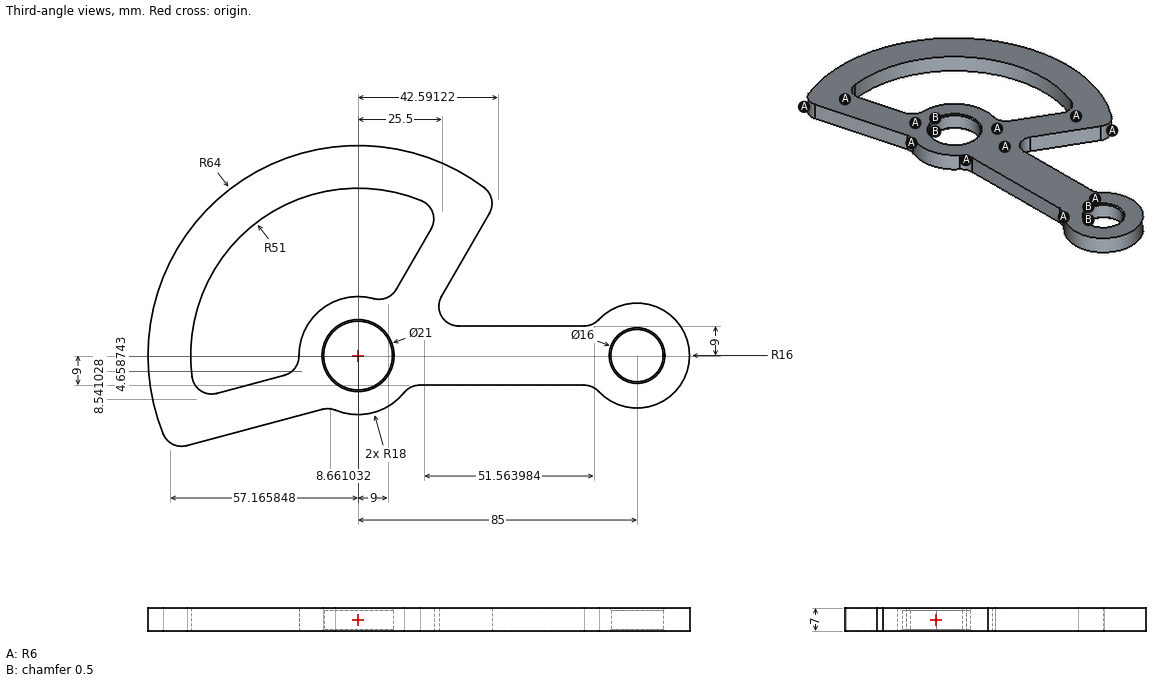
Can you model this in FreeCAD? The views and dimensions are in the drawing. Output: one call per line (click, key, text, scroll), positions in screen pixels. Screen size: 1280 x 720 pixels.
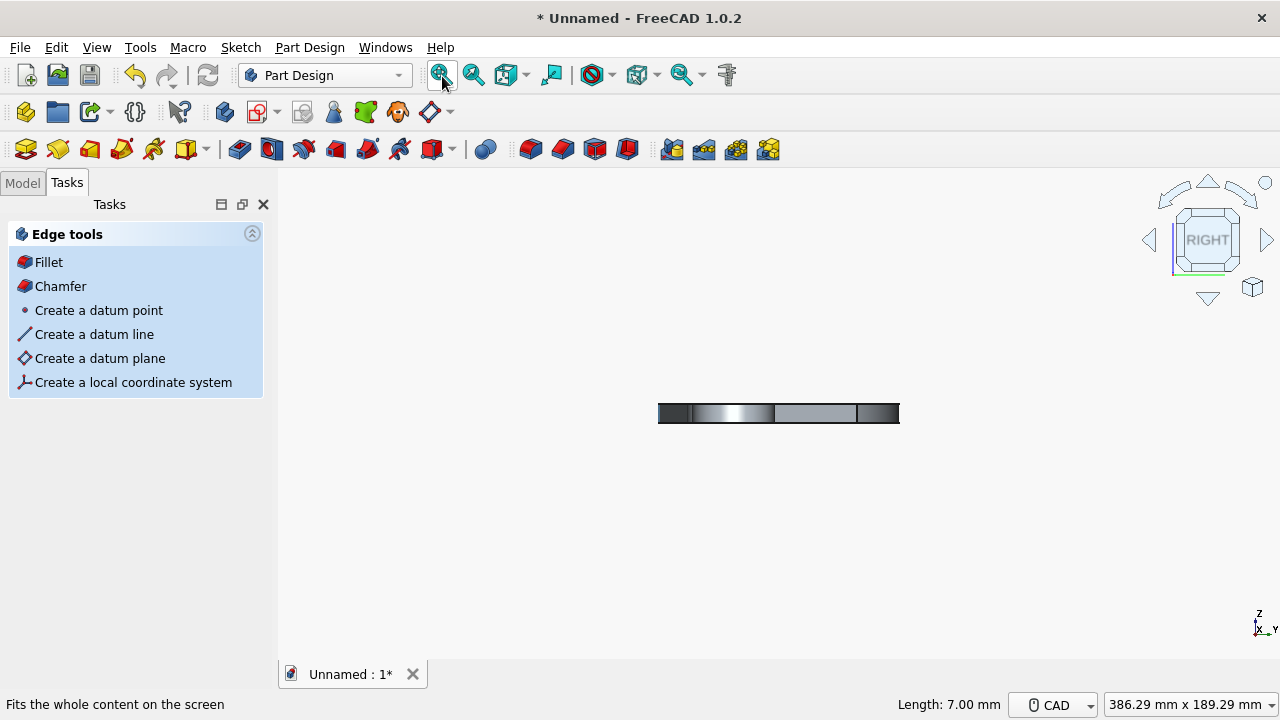
click(857, 412, ctrl)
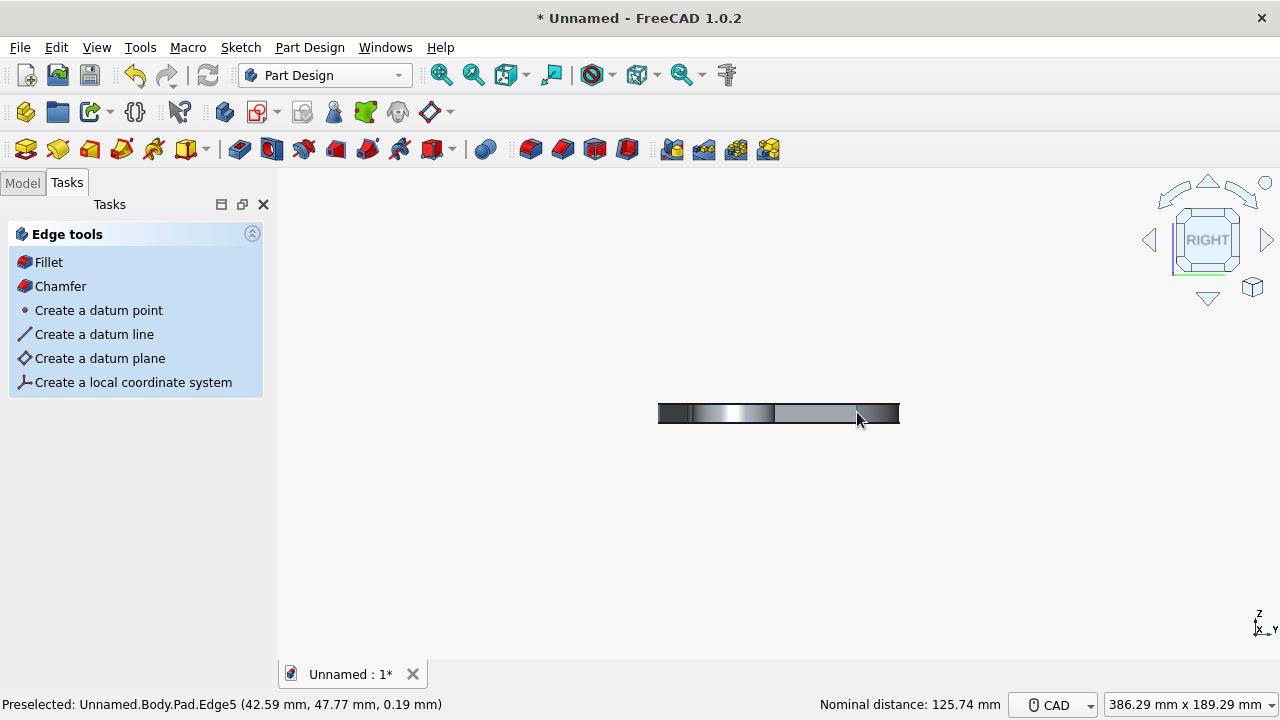
scroll(710, 412, up, 4)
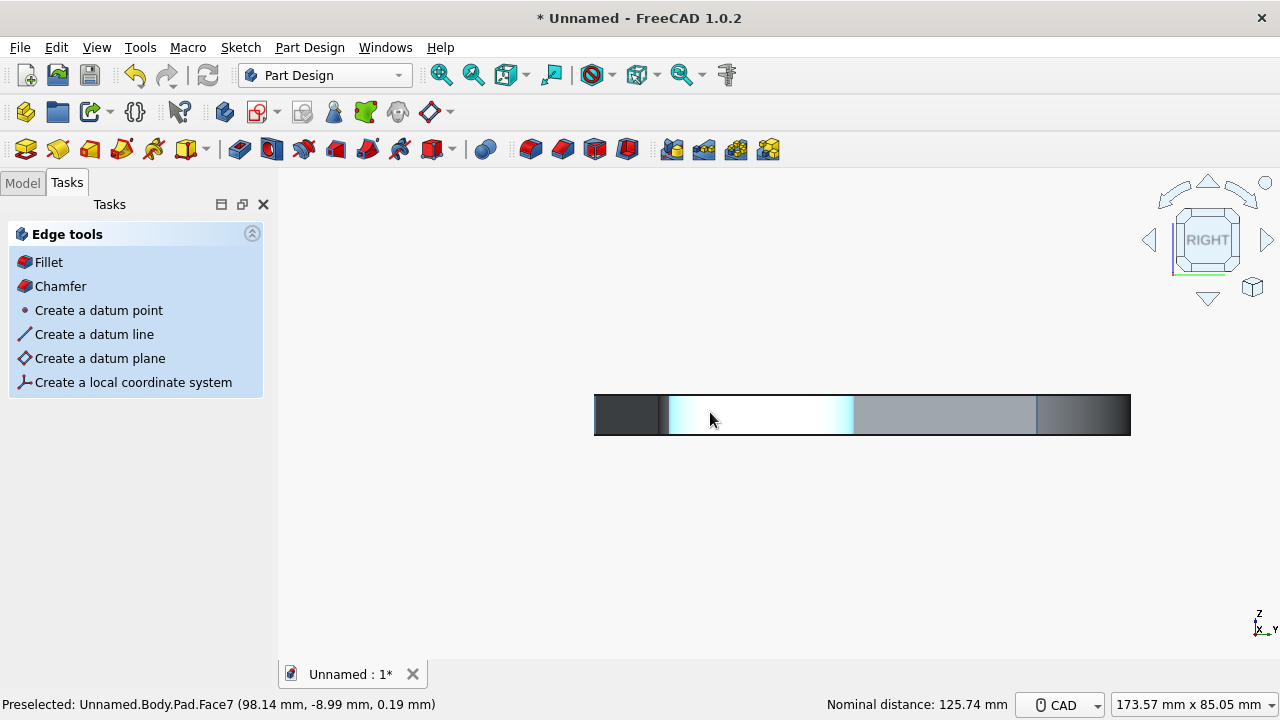
click(442, 76)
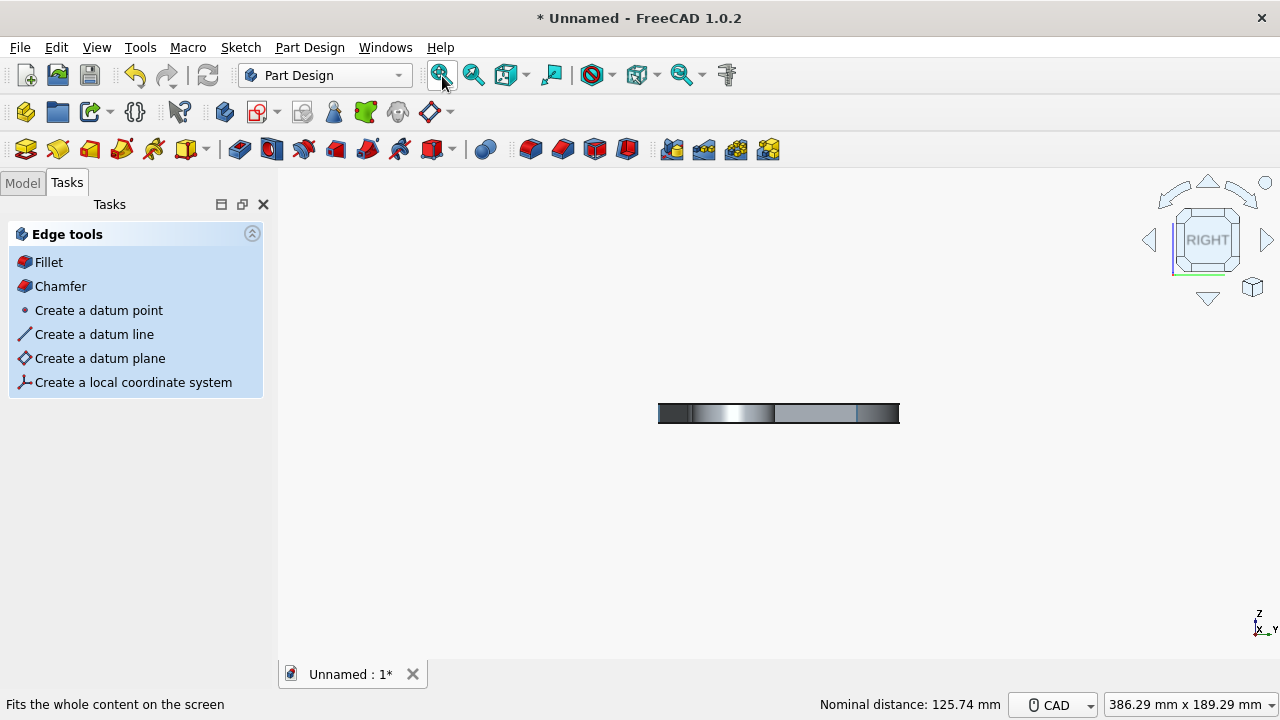
key(5)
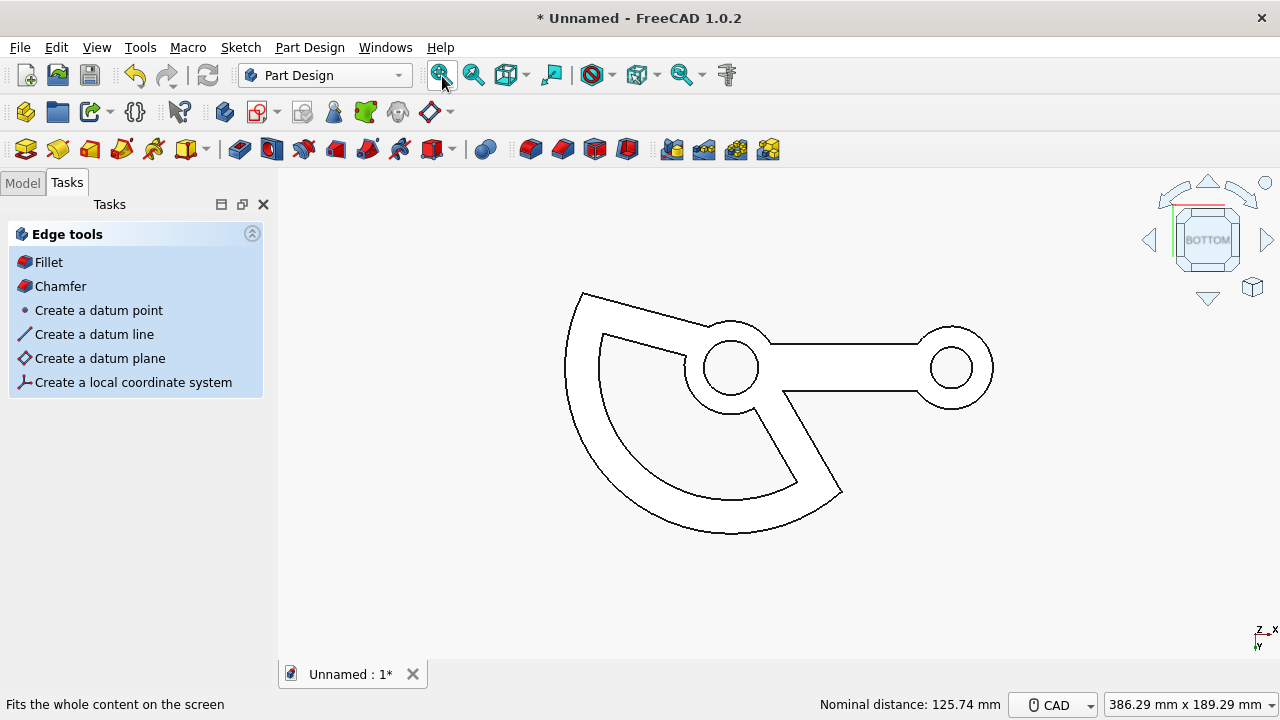
scroll(917, 343, up, 4)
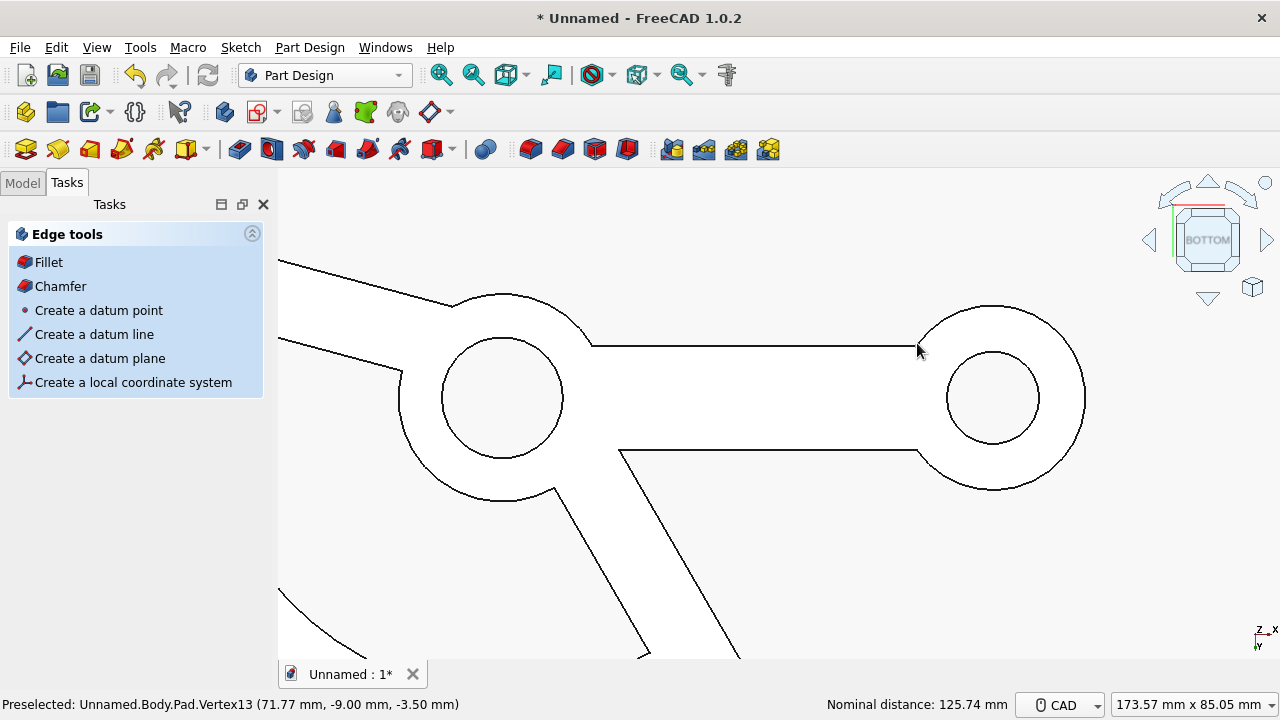
click(442, 76)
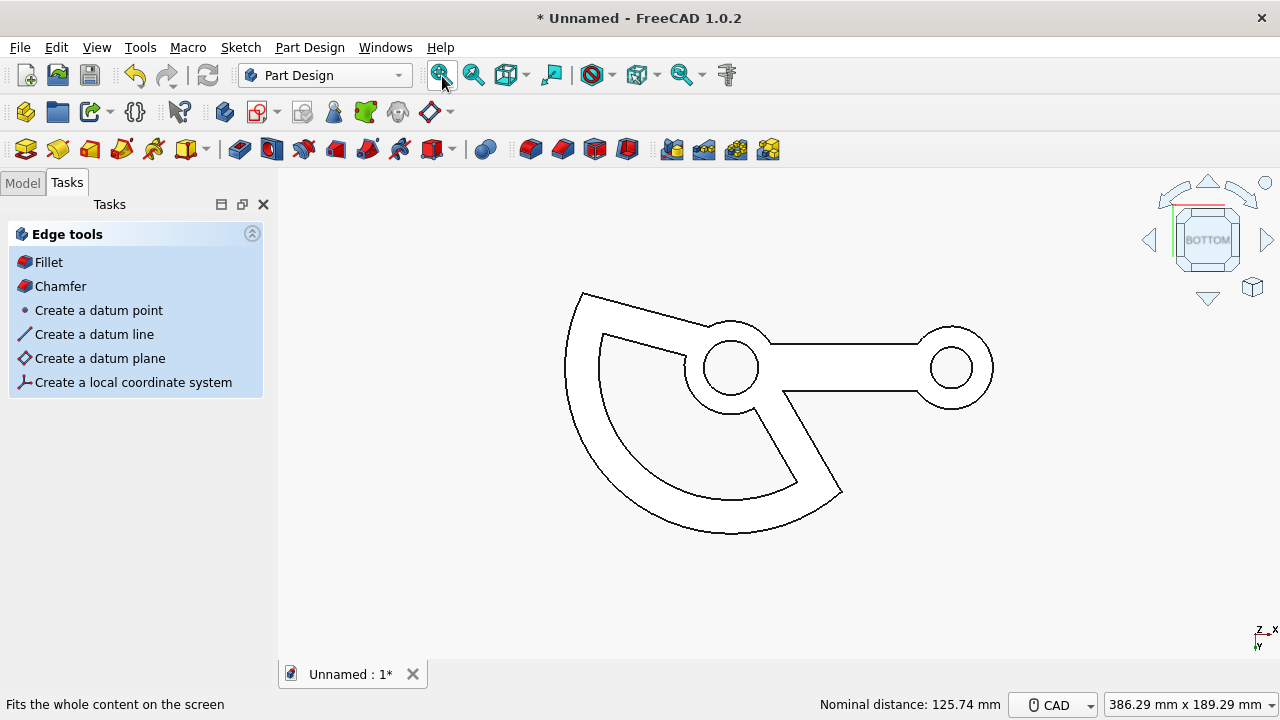
key(4)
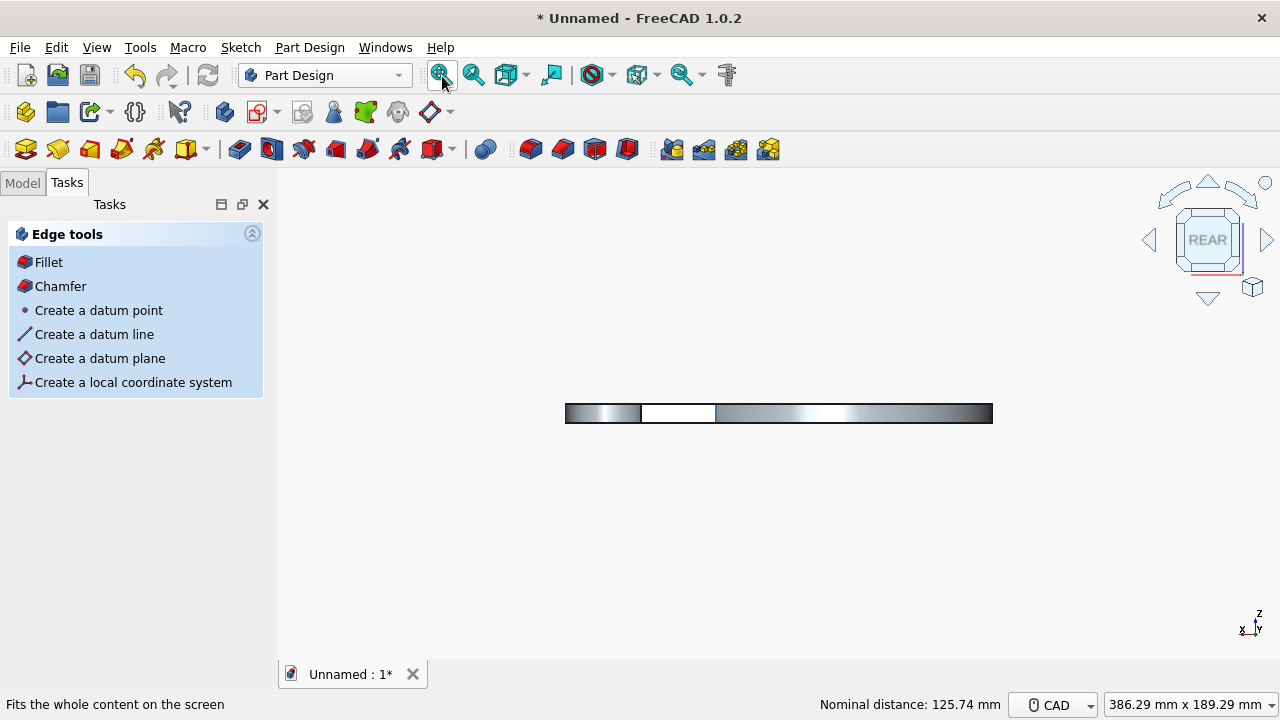
key(v)
key(f)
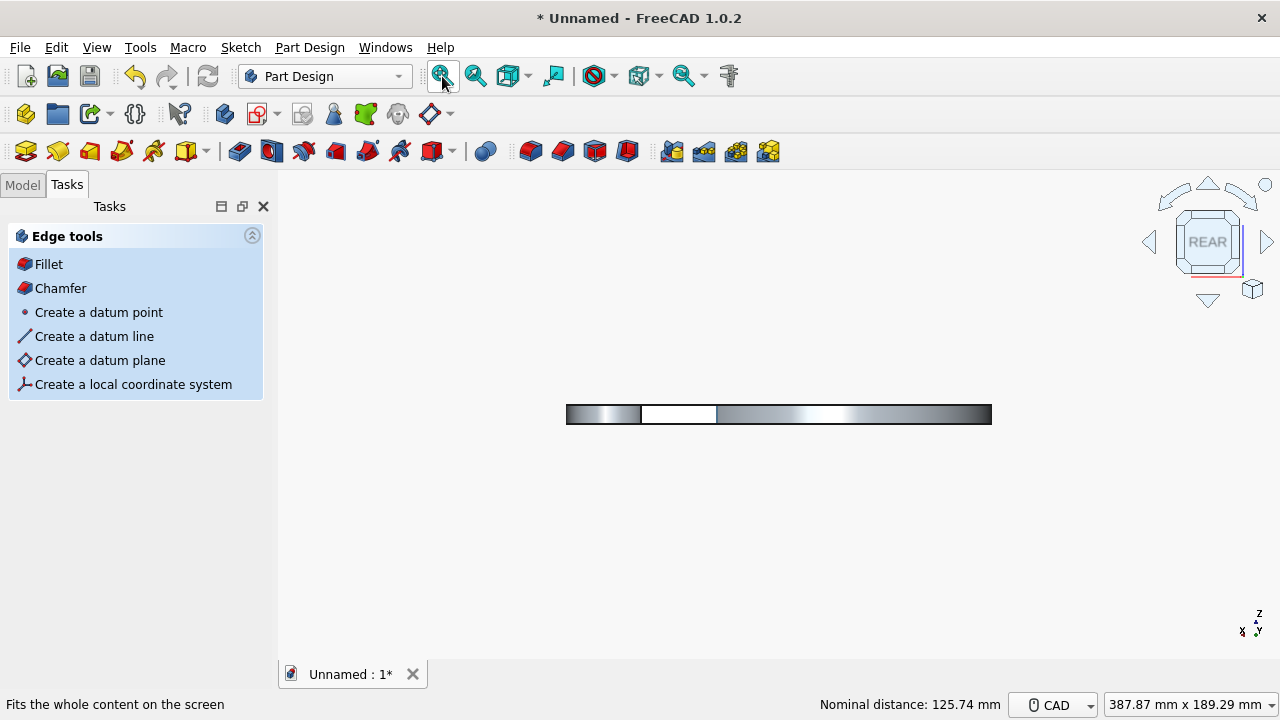
scroll(641, 414, up, 4)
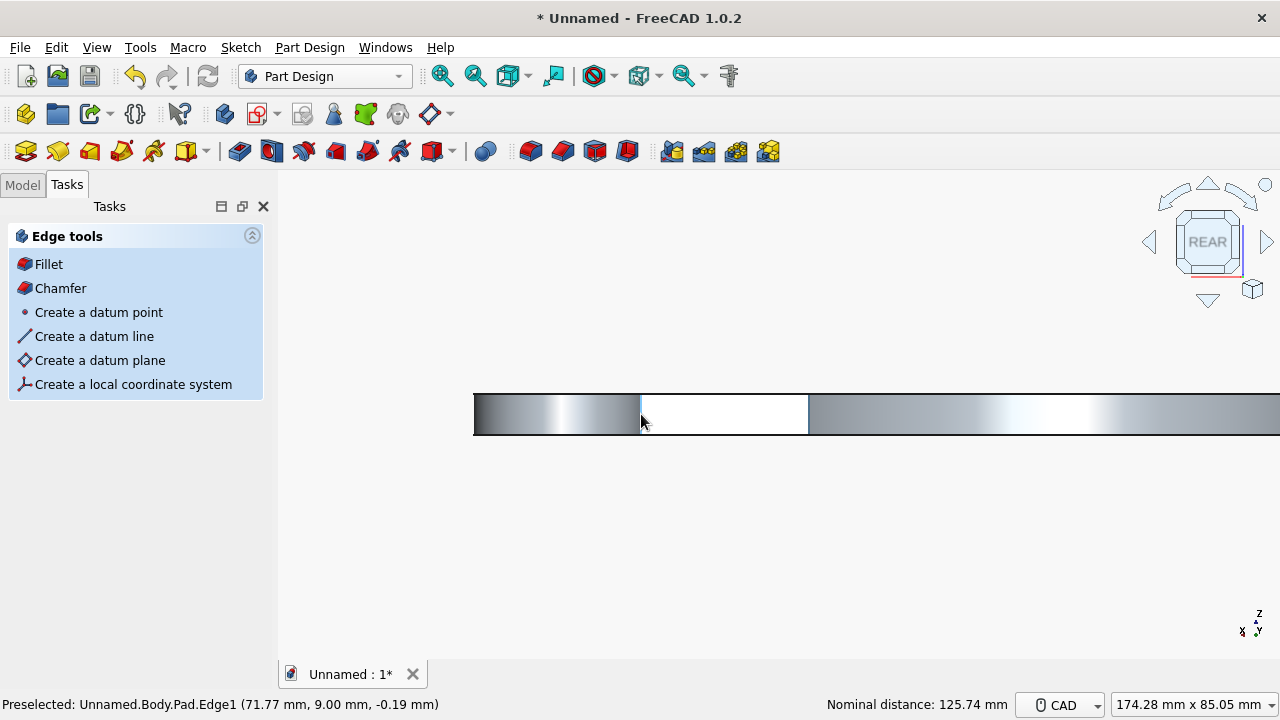
key(v)
key(f)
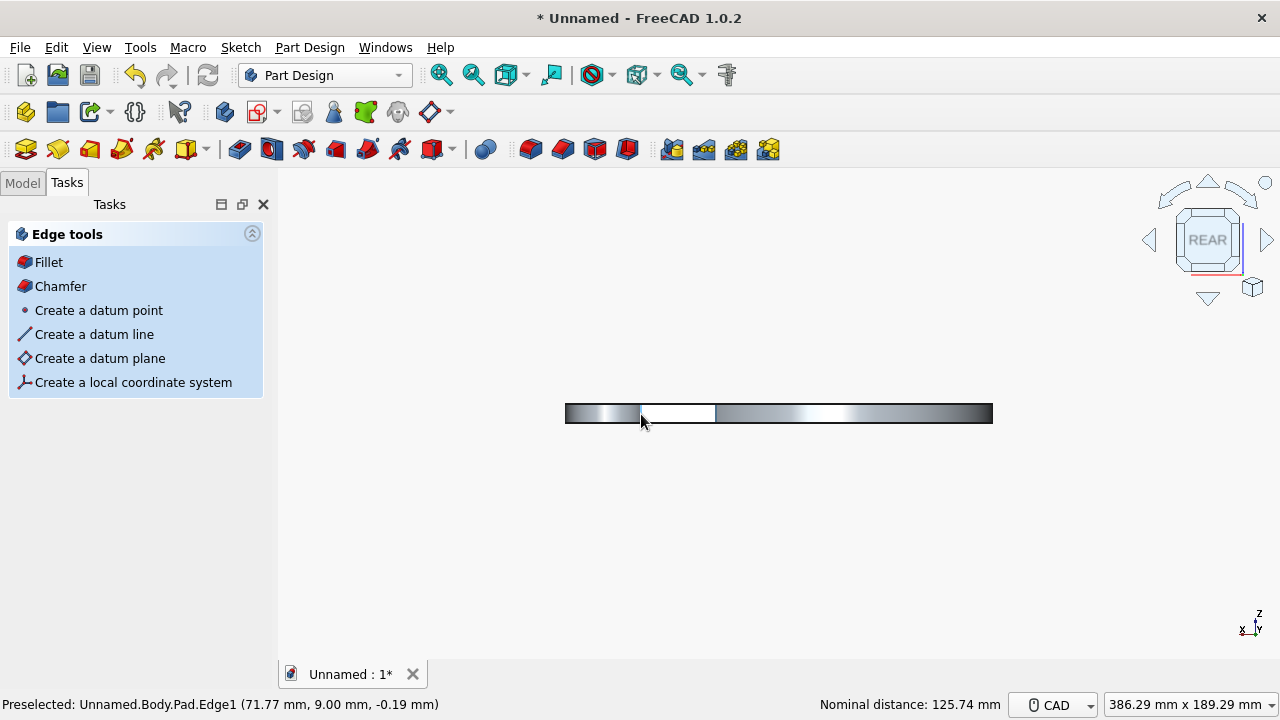
key(6)